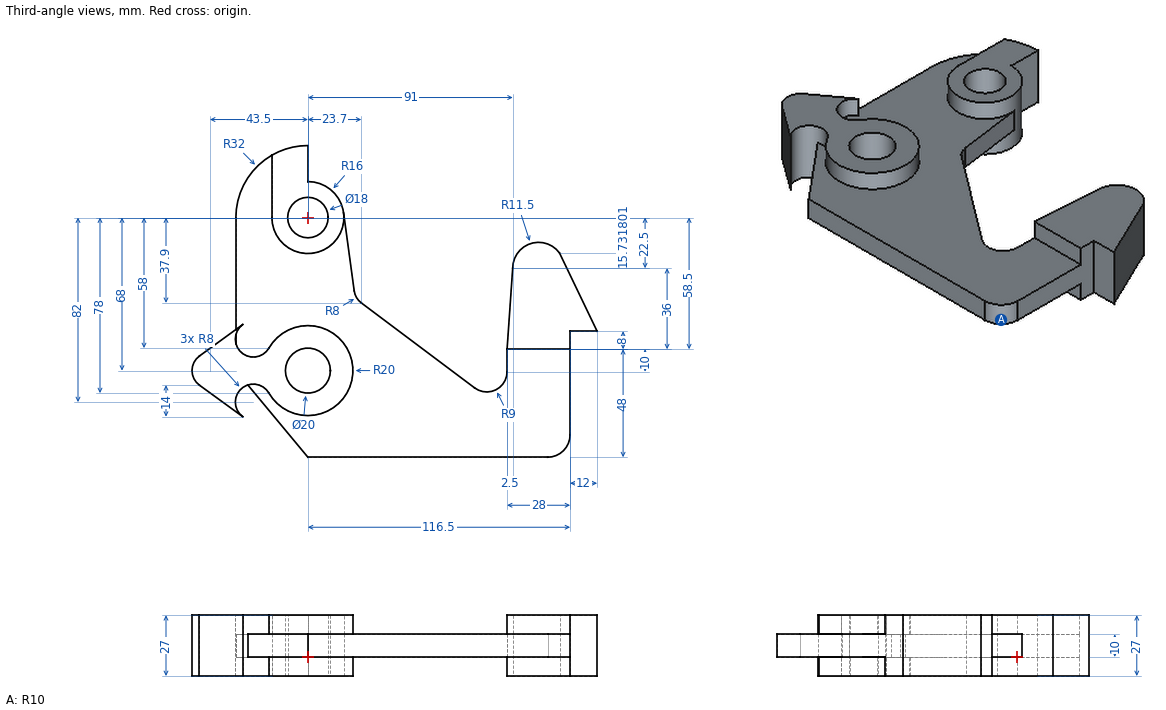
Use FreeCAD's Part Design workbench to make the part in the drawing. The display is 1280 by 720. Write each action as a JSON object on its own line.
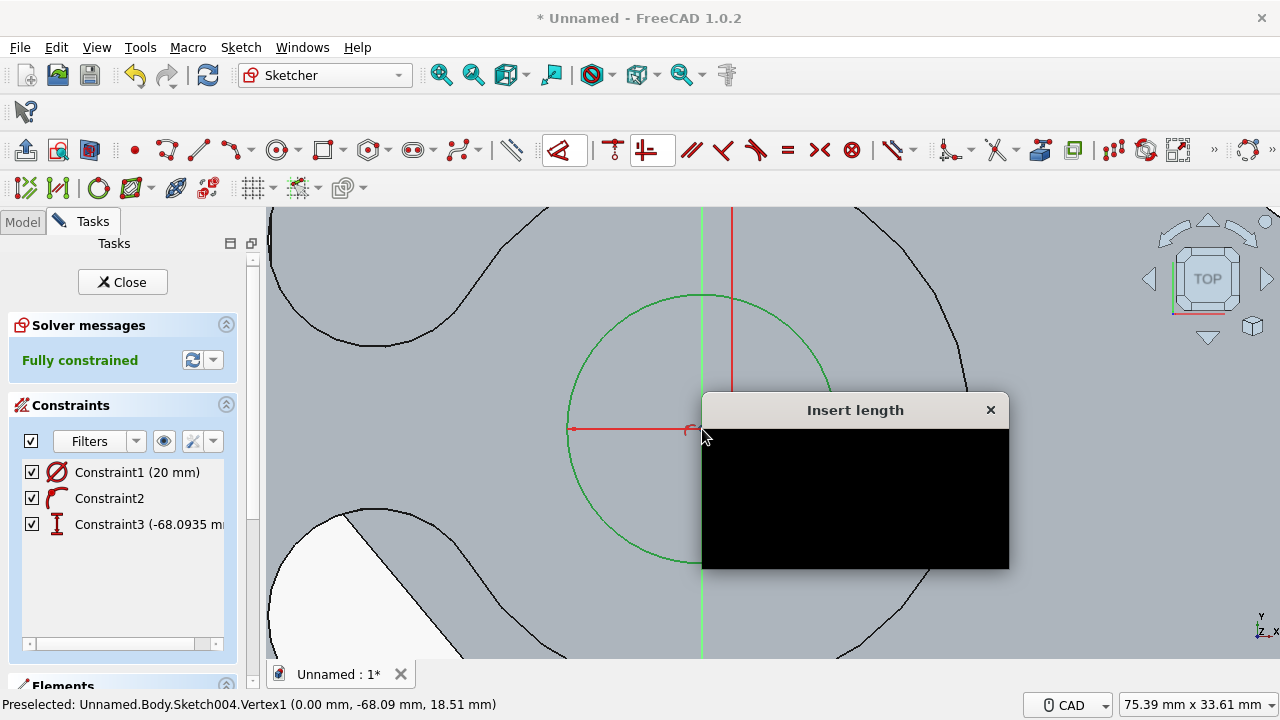
{"action": "type", "text": "-68"}
{"action": "key", "text": "Return"}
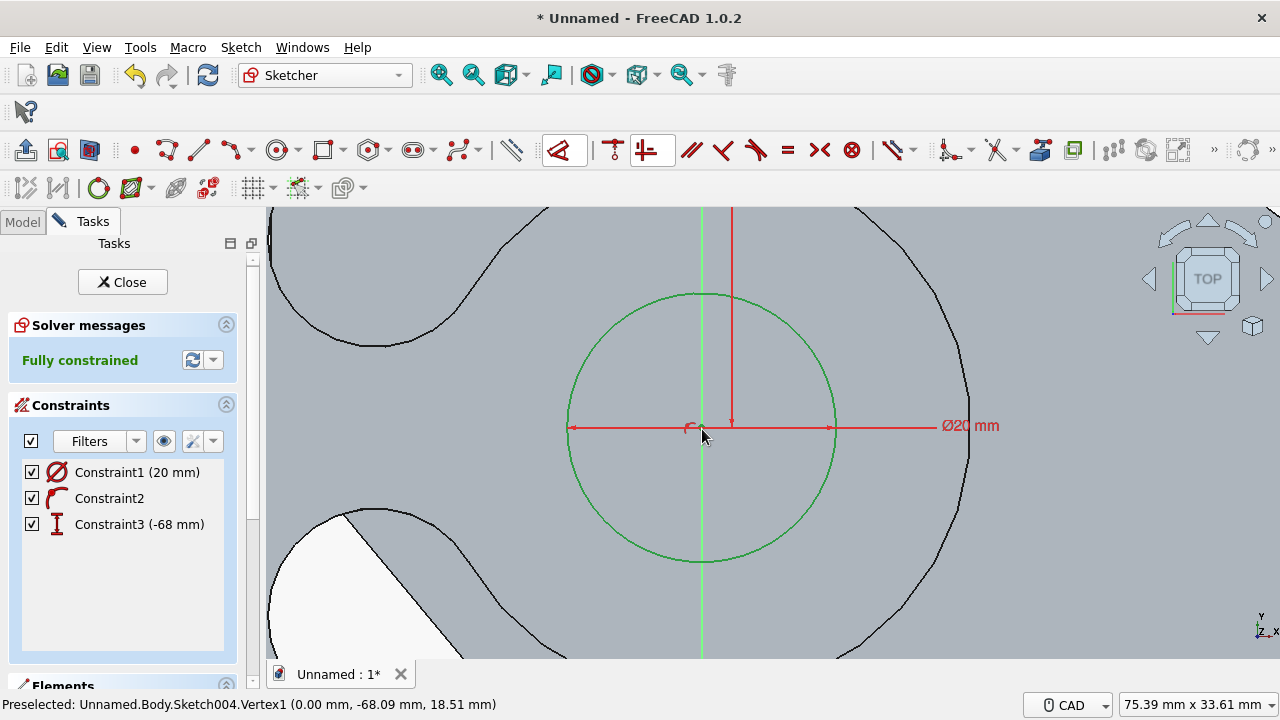
{"action": "left_click", "coordinate": [123, 282]}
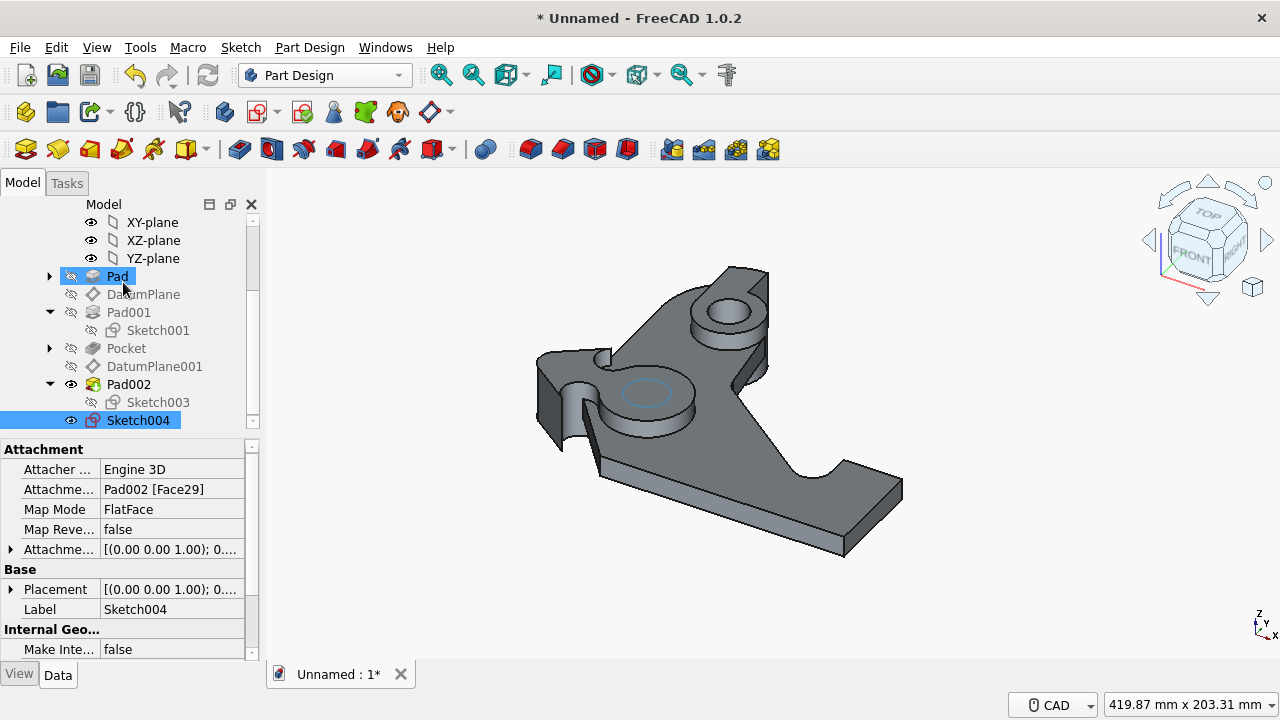
{"action": "left_click", "coordinate": [240, 150]}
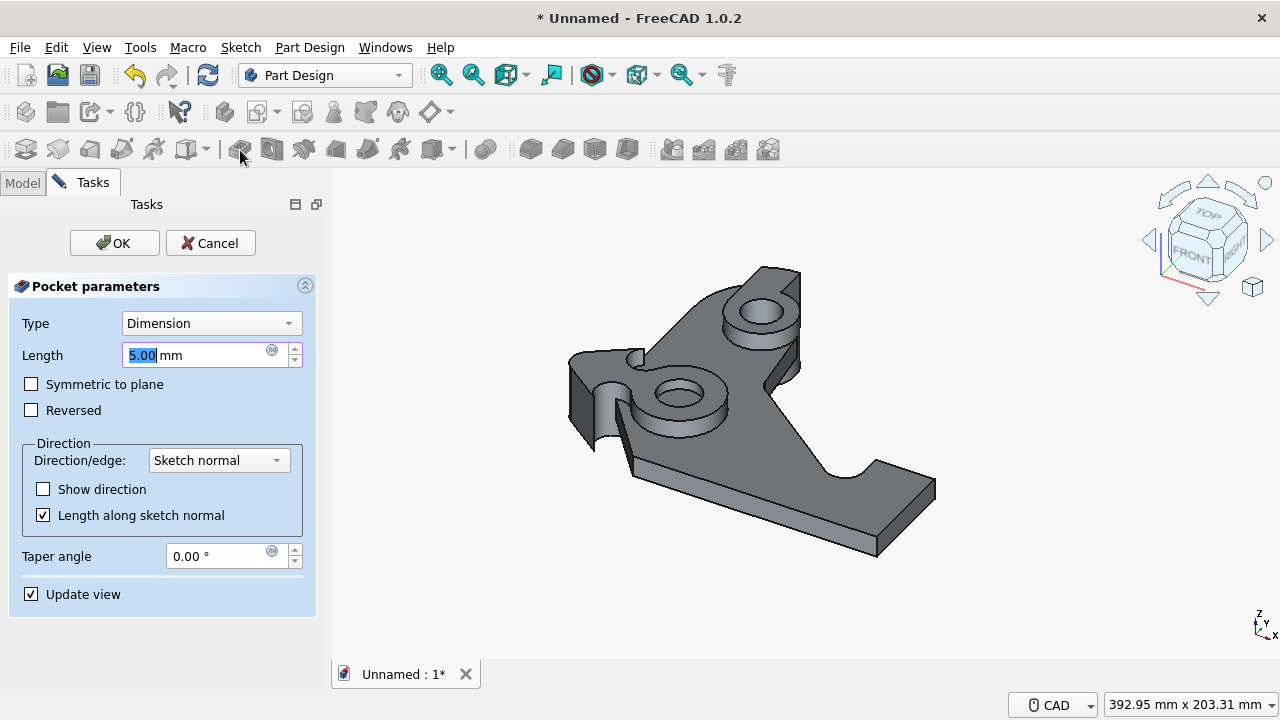
{"action": "type", "text": "27"}
{"action": "key", "text": "Tab"}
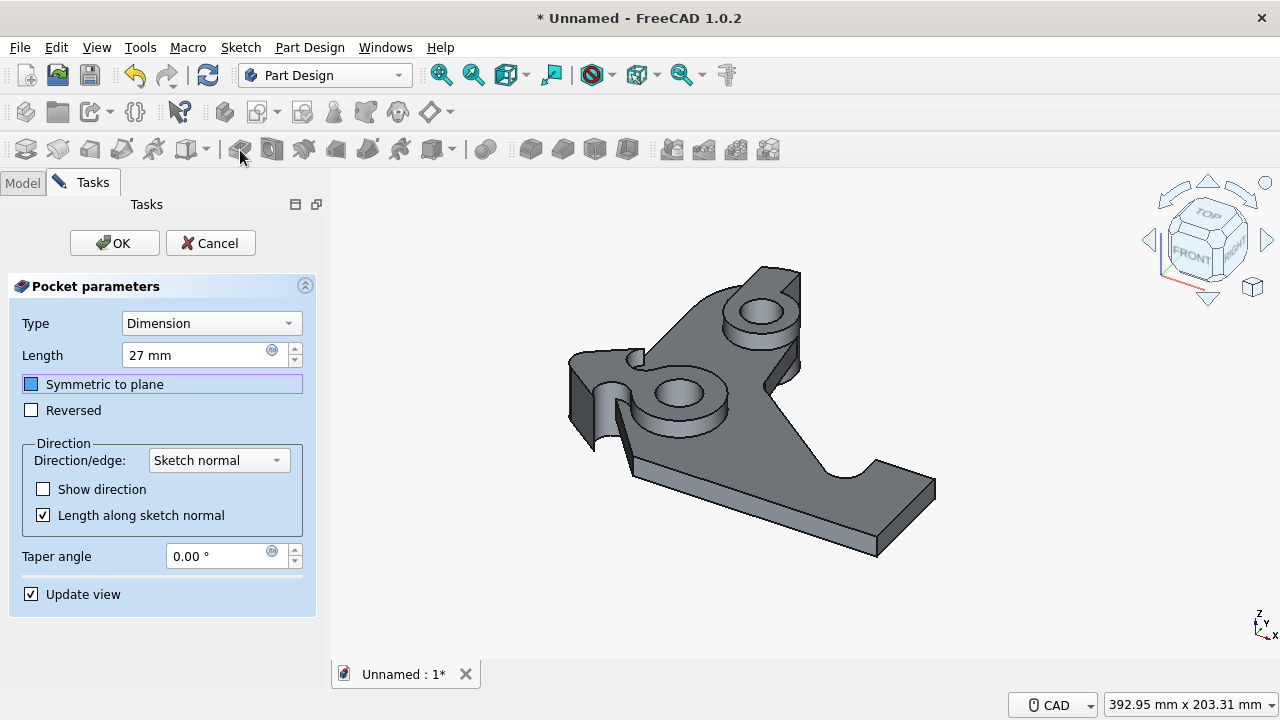
{"action": "left_click", "coordinate": [115, 243]}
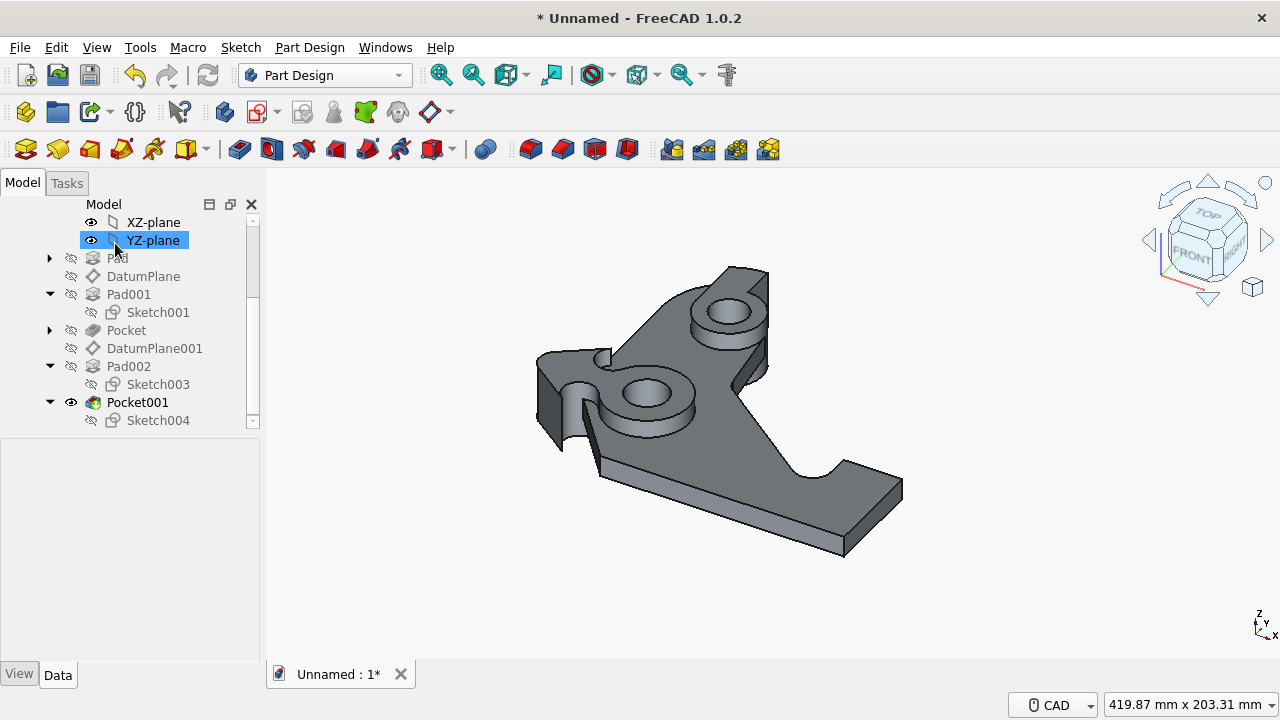
{"action": "scroll", "coordinate": [160, 326], "scroll_direction": "down", "scroll_amount": 3}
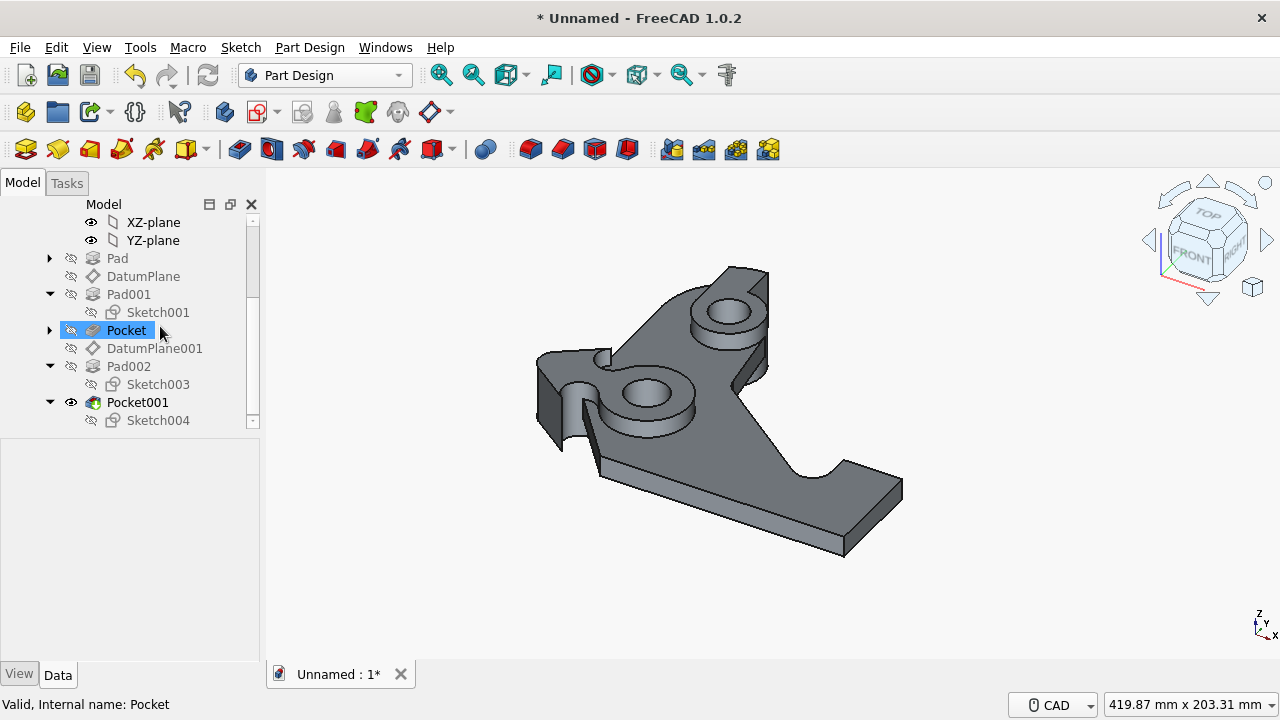
{"action": "scroll", "coordinate": [160, 326], "scroll_direction": "up", "scroll_amount": 15}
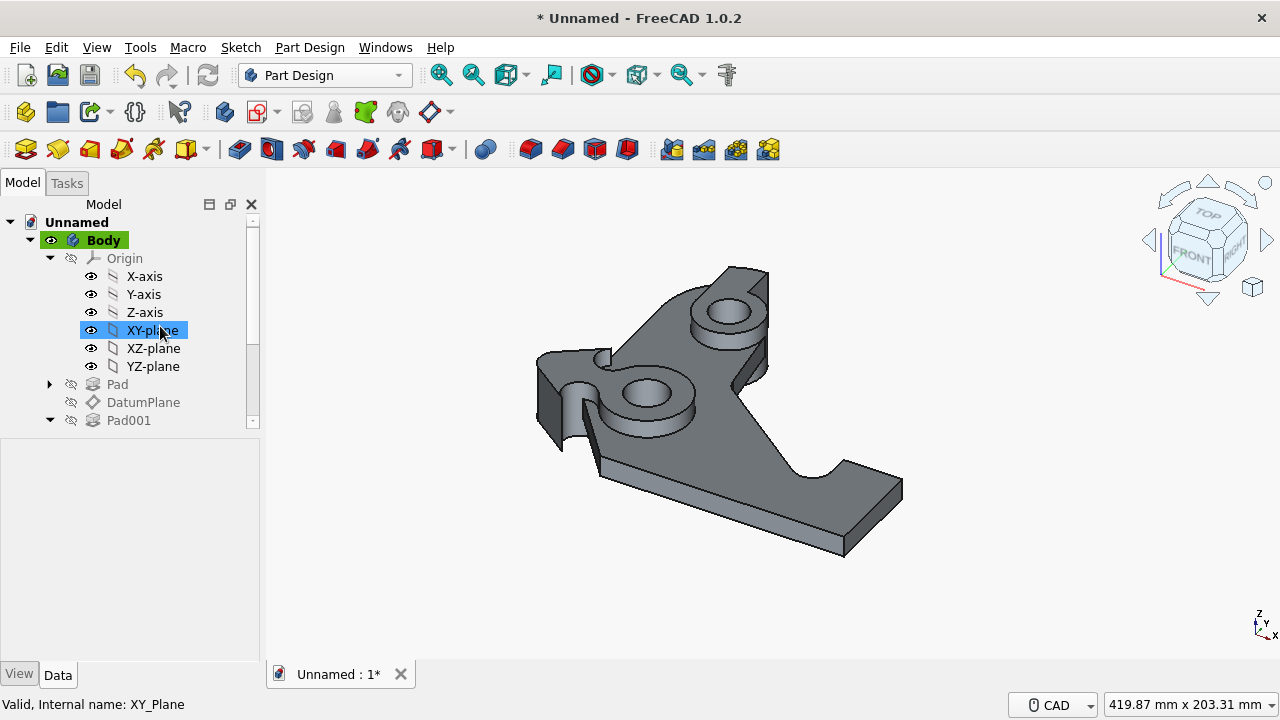
{"action": "left_click", "coordinate": [136, 330]}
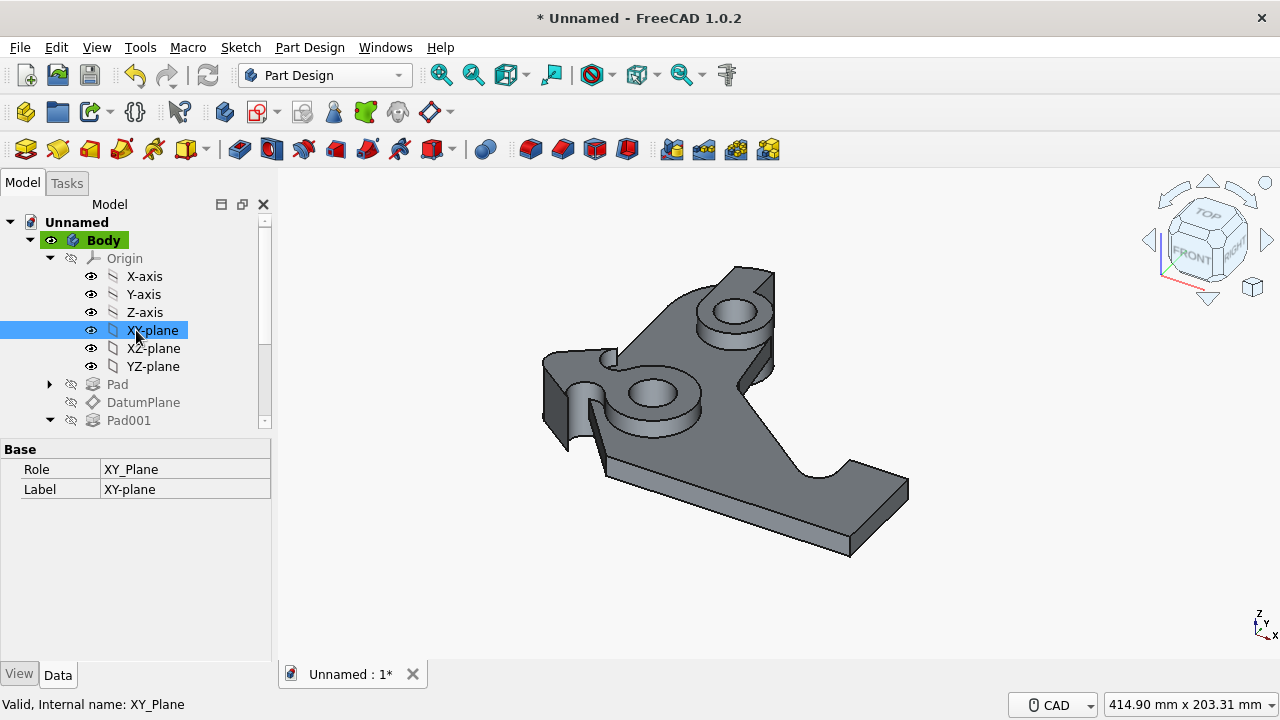
{"action": "left_click", "coordinate": [430, 112]}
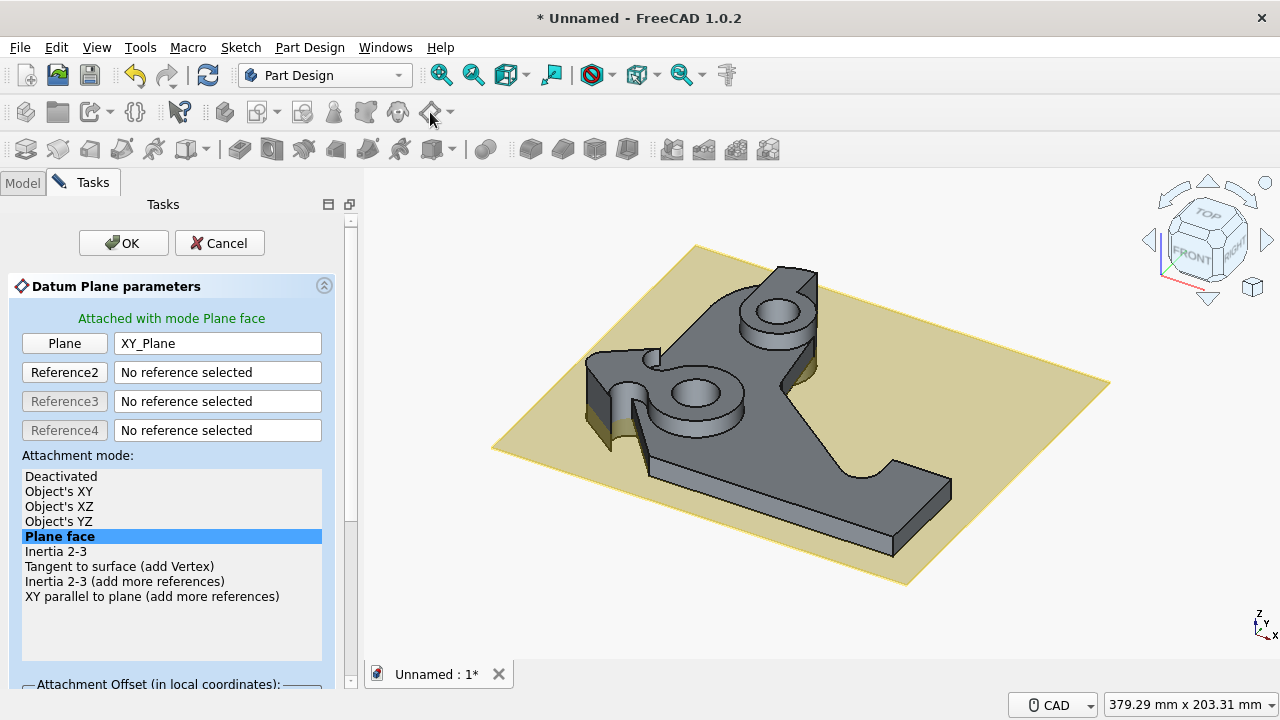
{"action": "scroll", "coordinate": [351, 451], "scroll_direction": "down", "scroll_amount": 3}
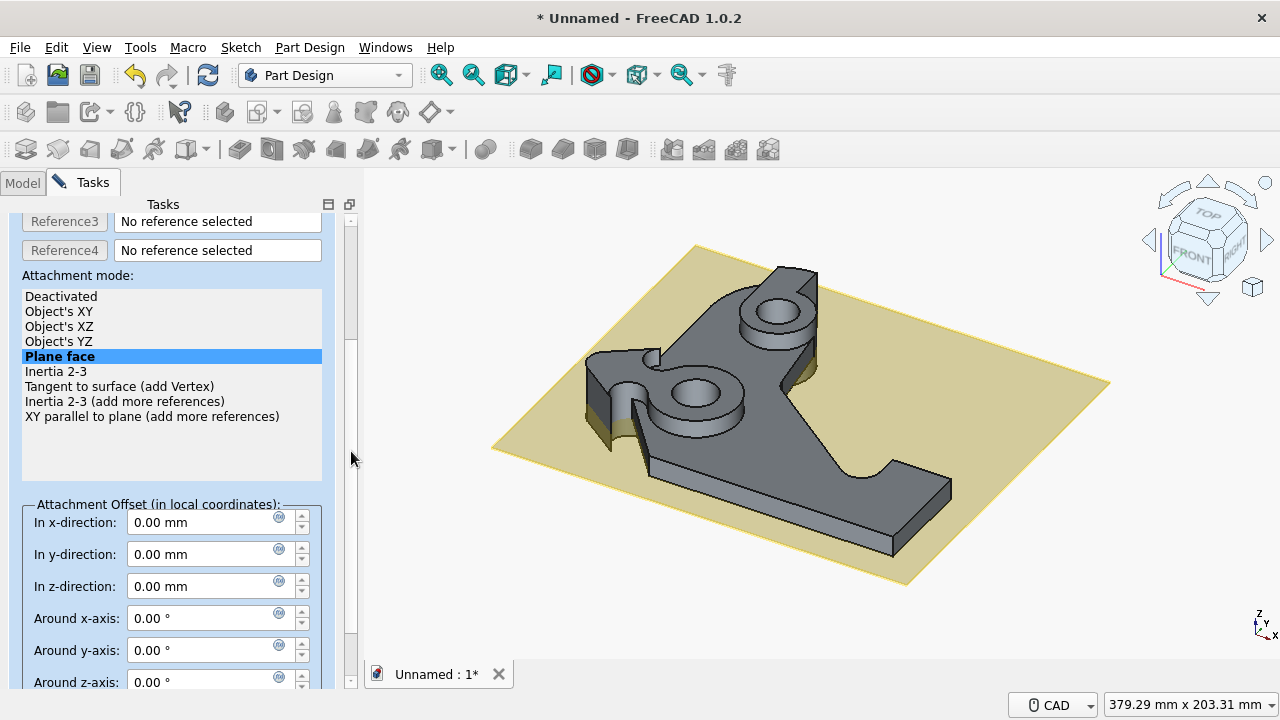
{"action": "triple_click", "coordinate": [210, 586]}